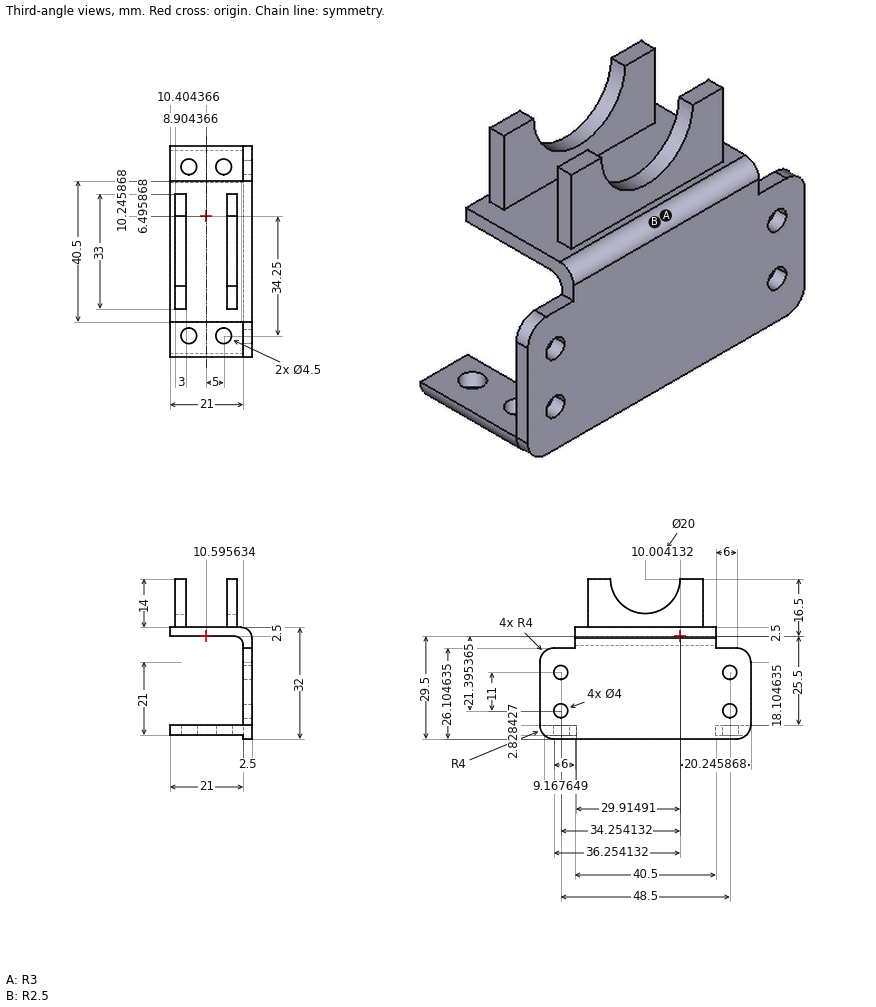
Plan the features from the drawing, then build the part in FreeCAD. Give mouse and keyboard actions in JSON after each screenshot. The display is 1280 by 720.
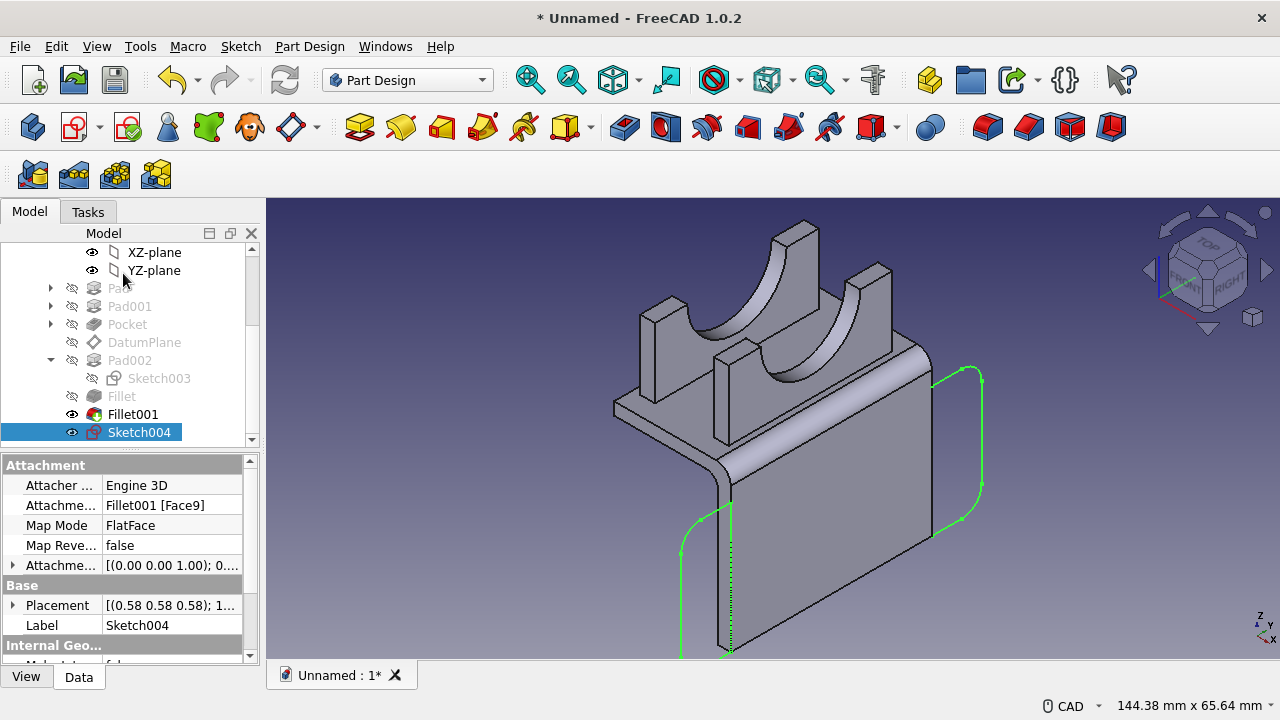
{"action": "left_click", "coordinate": [360, 128]}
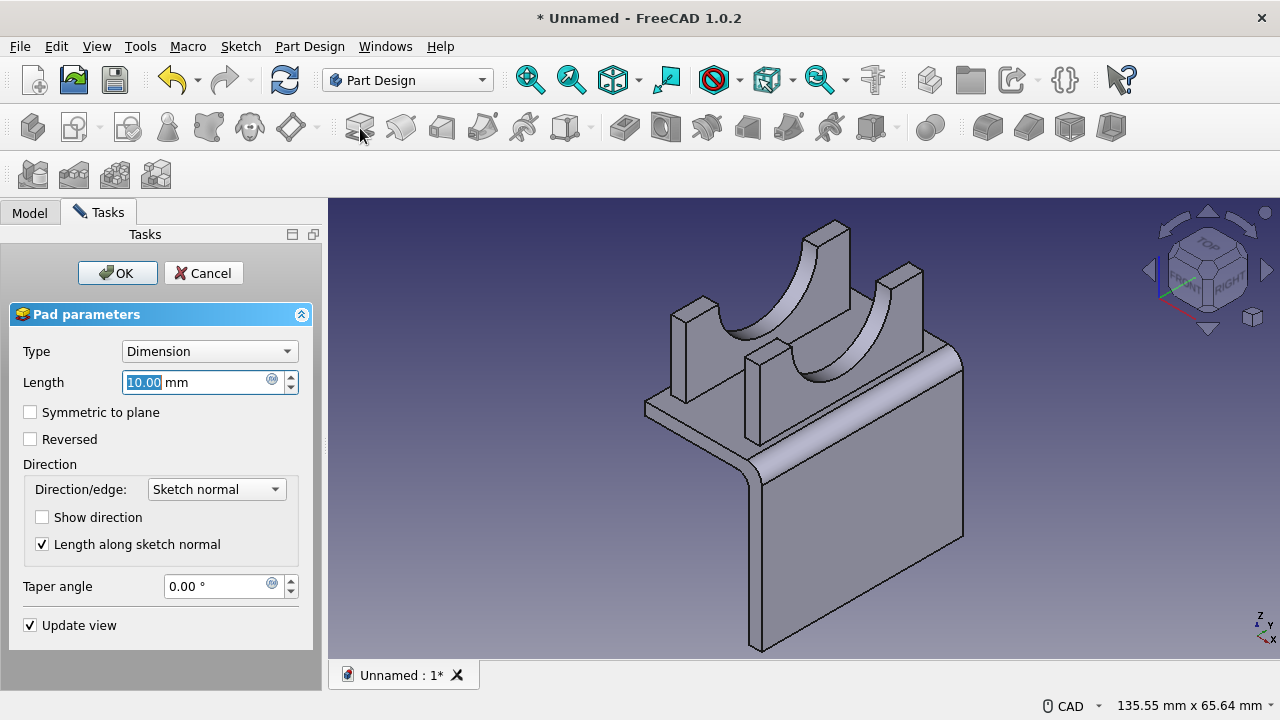
{"action": "type", "text": "2.5"}
{"action": "key", "text": "Tab"}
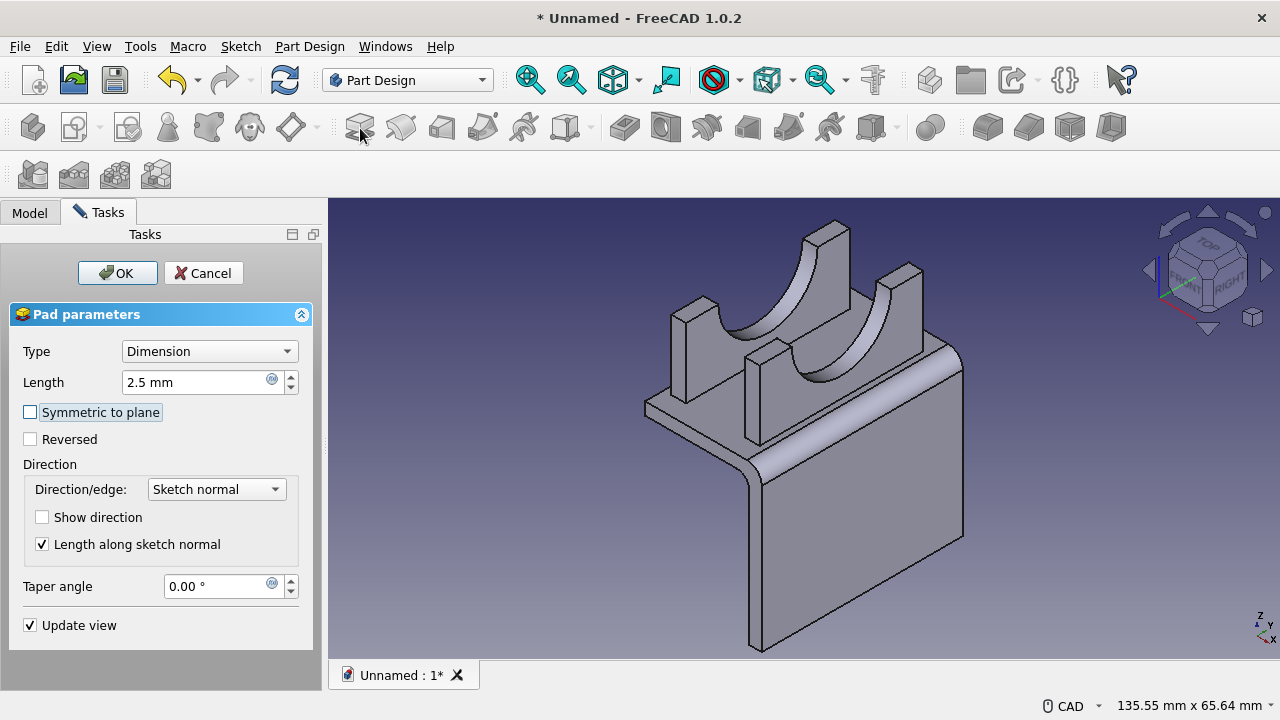
{"action": "left_click", "coordinate": [31, 439]}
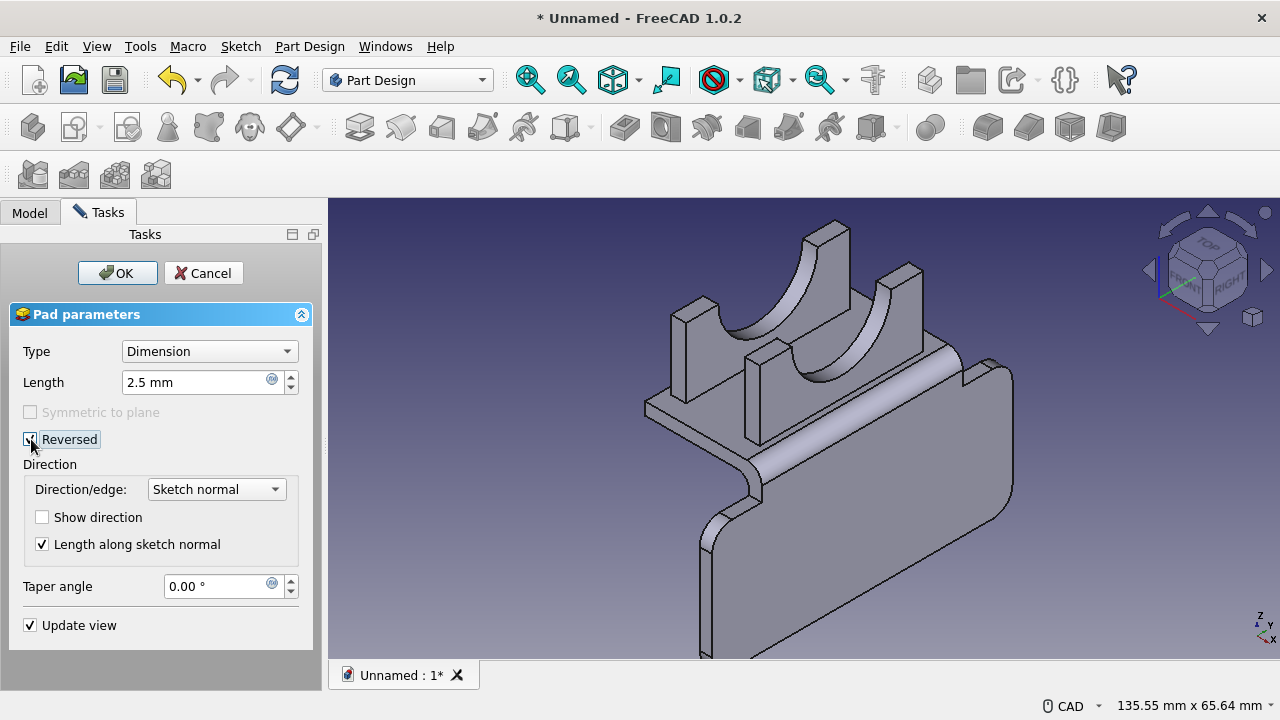
{"action": "left_click", "coordinate": [118, 273]}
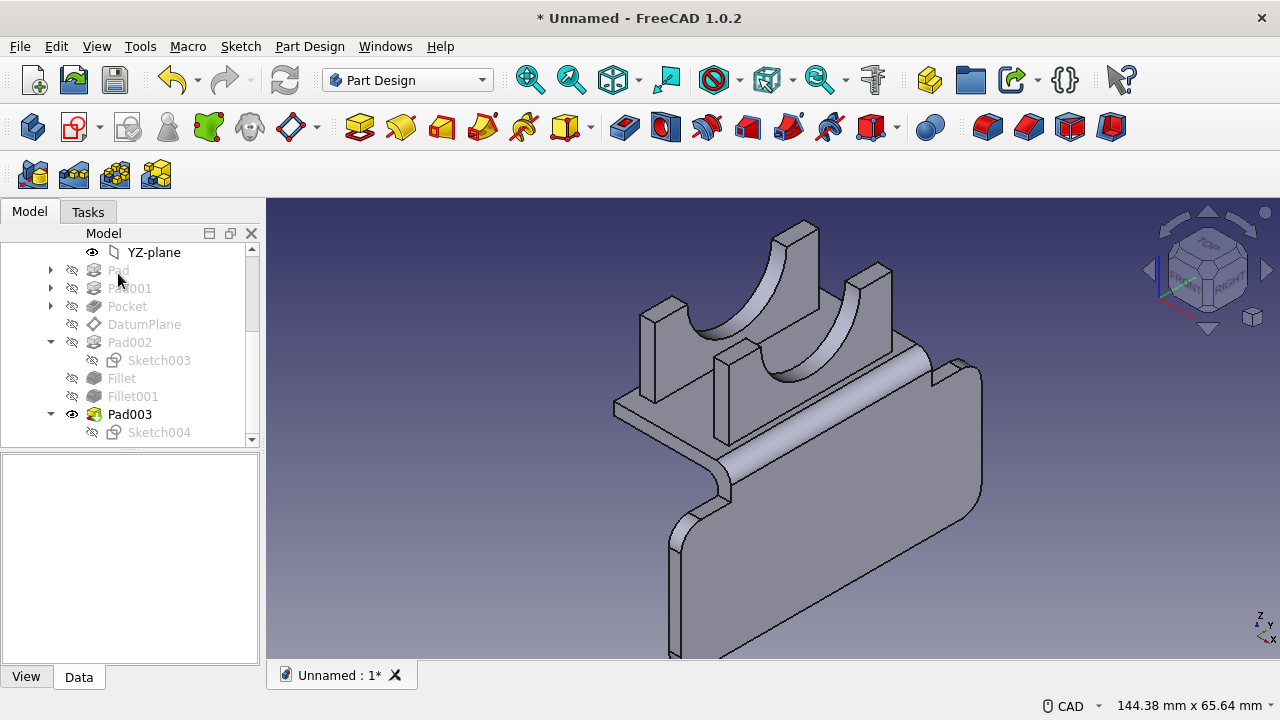
{"action": "left_click", "coordinate": [531, 80]}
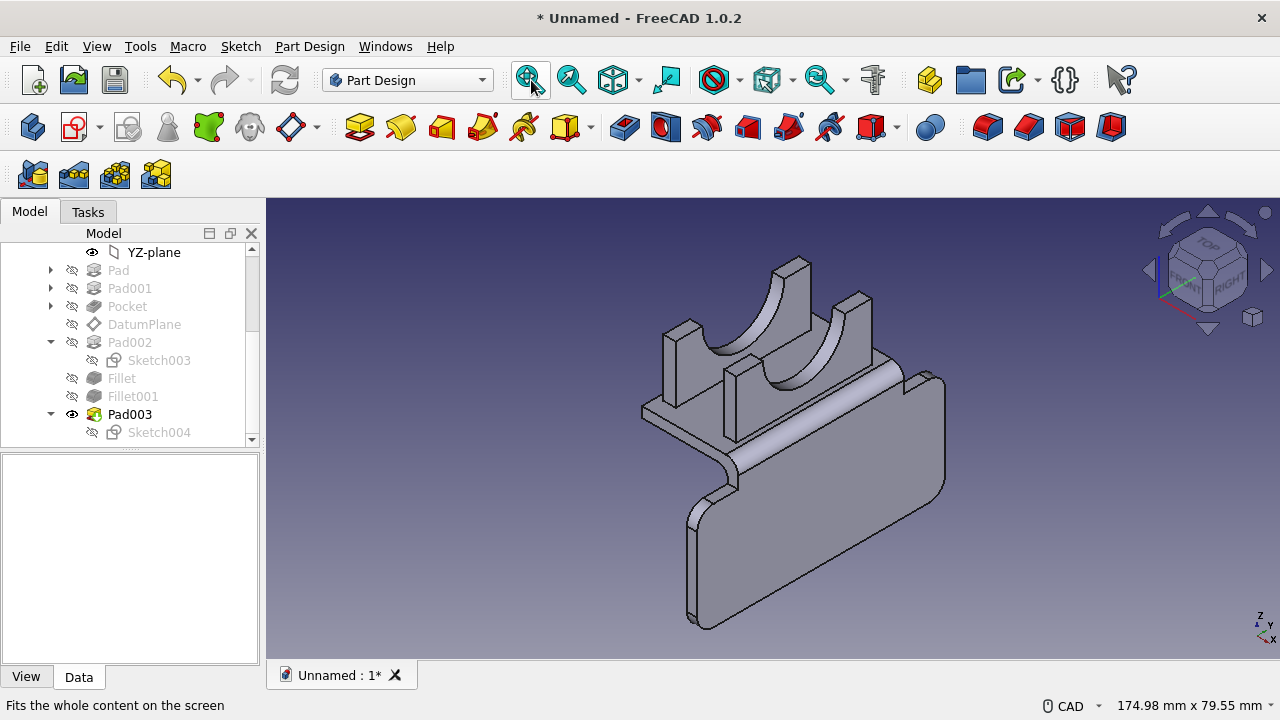
{"action": "left_click", "coordinate": [786, 516]}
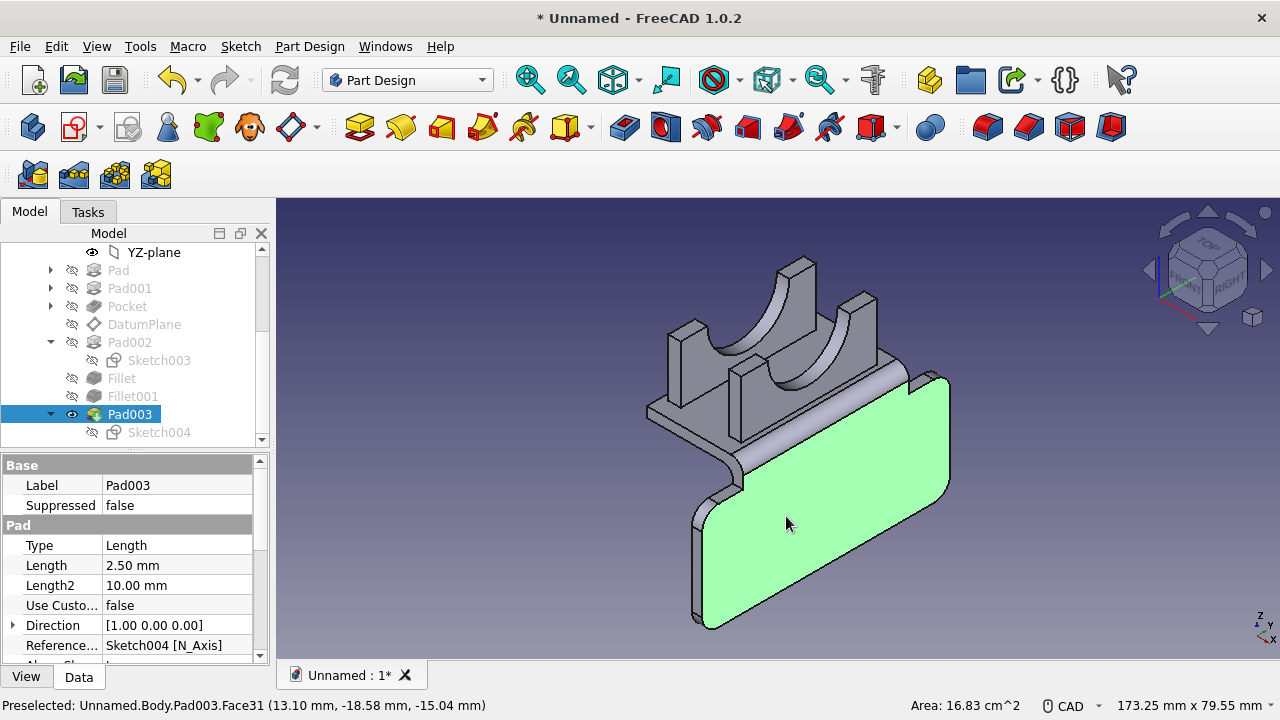
{"action": "left_click", "coordinate": [74, 128]}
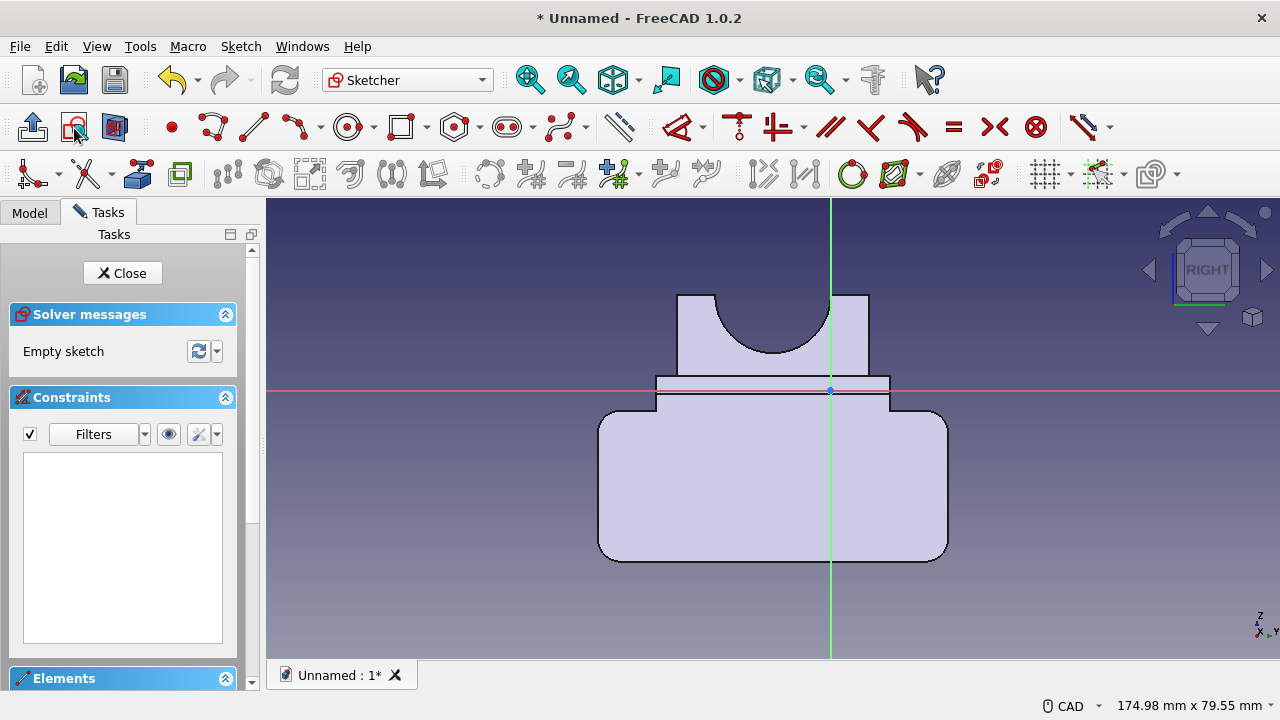
{"action": "scroll", "coordinate": [856, 495], "scroll_direction": "up", "scroll_amount": 3}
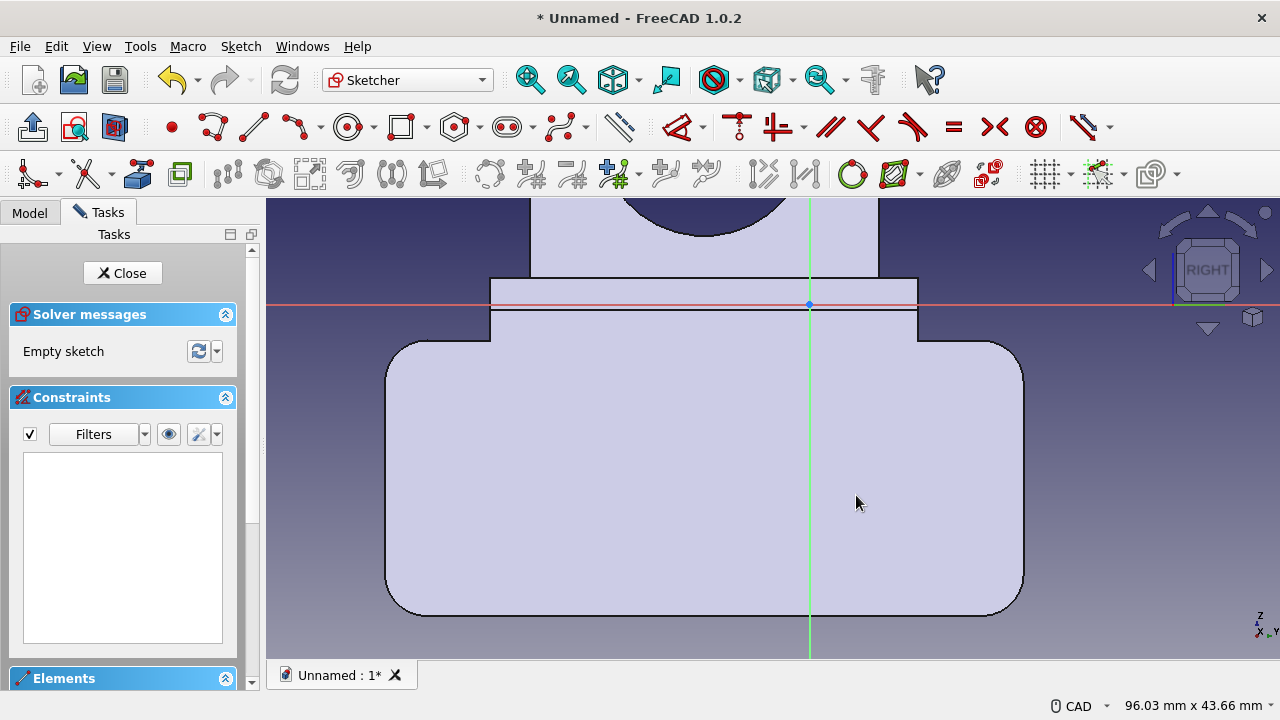
{"action": "left_click", "coordinate": [348, 128]}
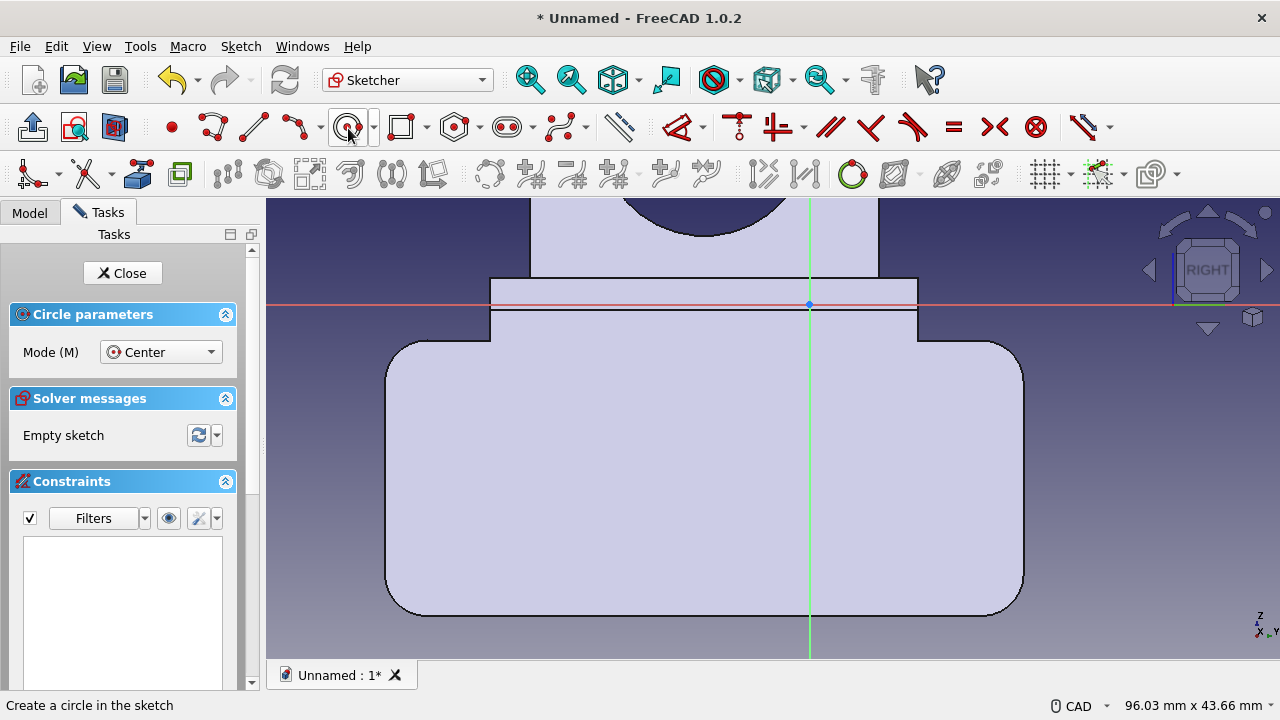
{"action": "left_click", "coordinate": [448, 531]}
{"action": "left_click", "coordinate": [463, 516]}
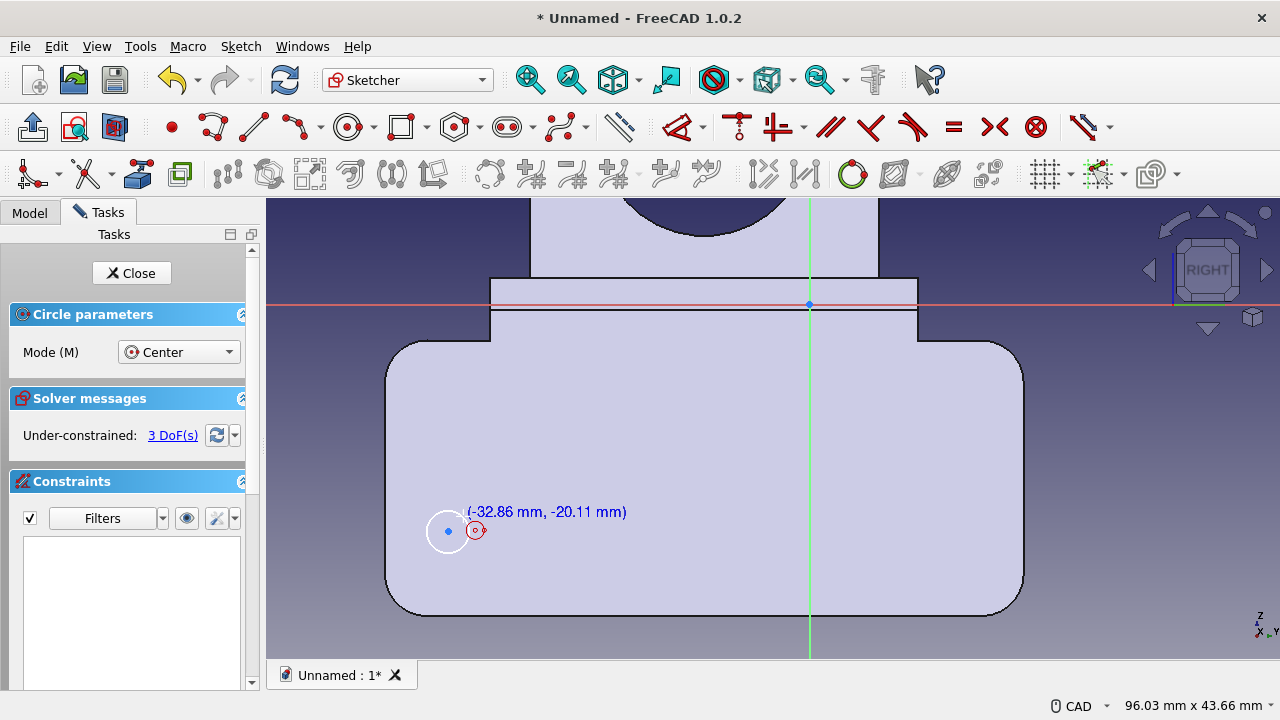
{"action": "left_click", "coordinate": [448, 414]}
{"action": "left_click", "coordinate": [463, 399]}